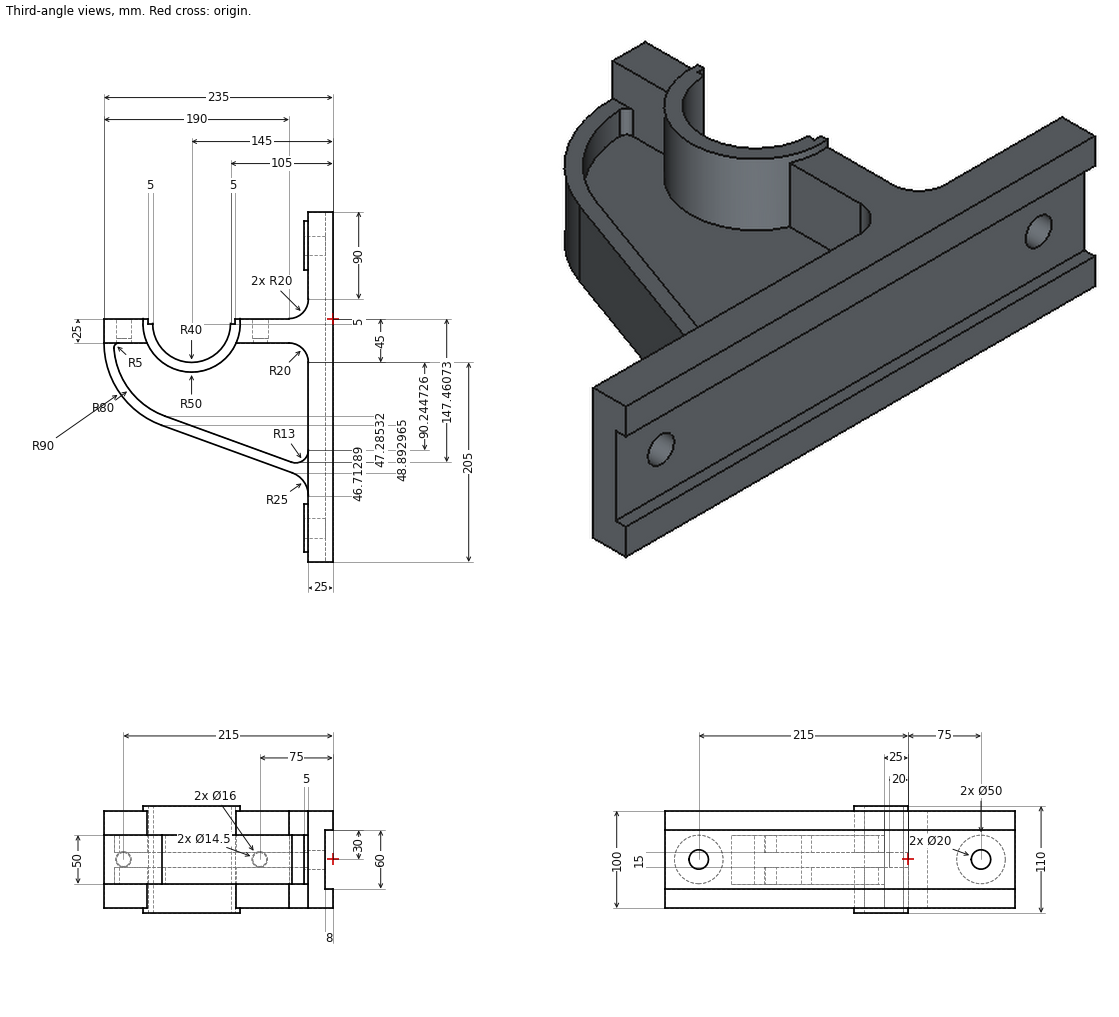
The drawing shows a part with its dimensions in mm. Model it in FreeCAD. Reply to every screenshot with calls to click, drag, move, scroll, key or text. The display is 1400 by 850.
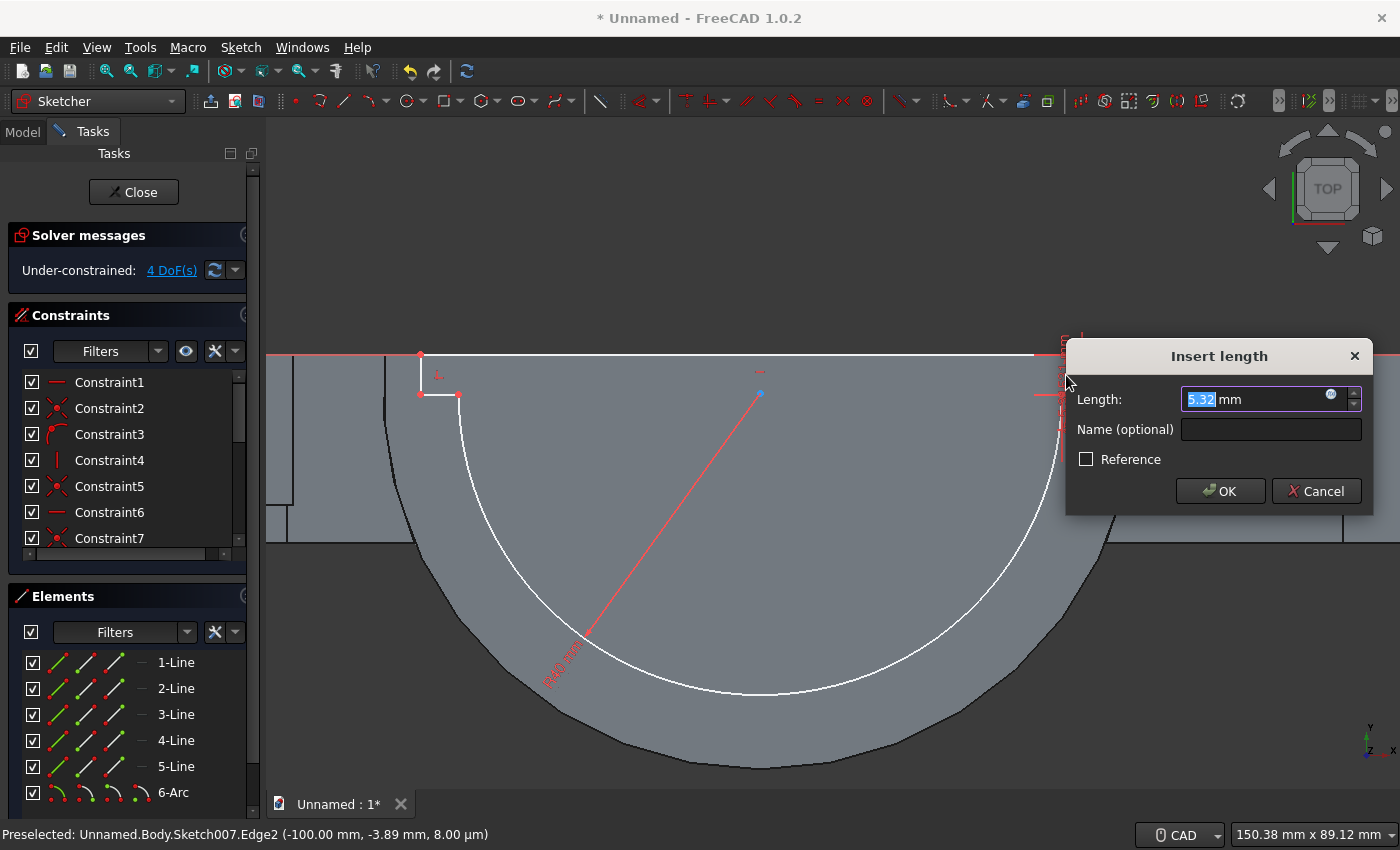
text(5)
key(Return)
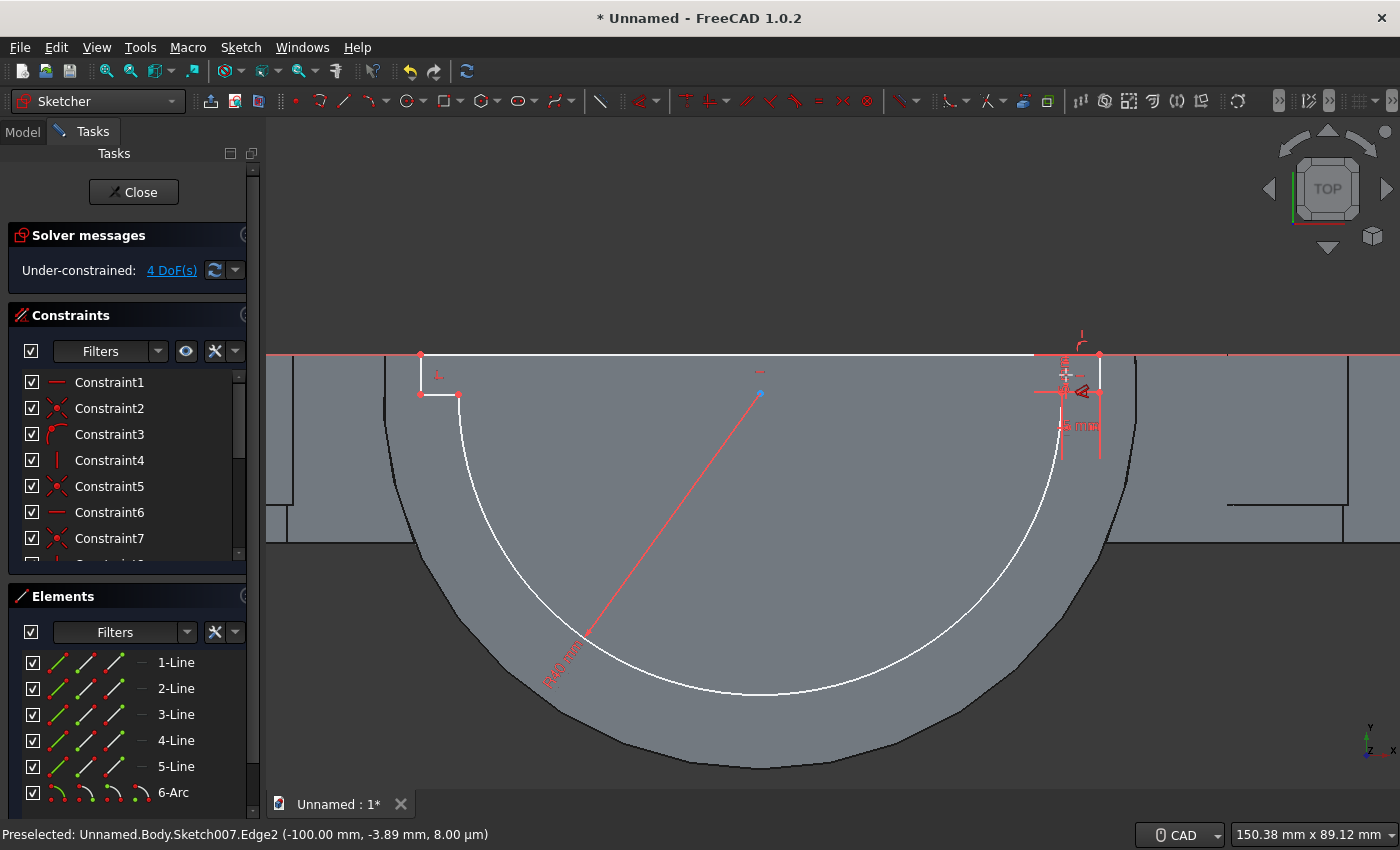
click(421, 367)
click(387, 375)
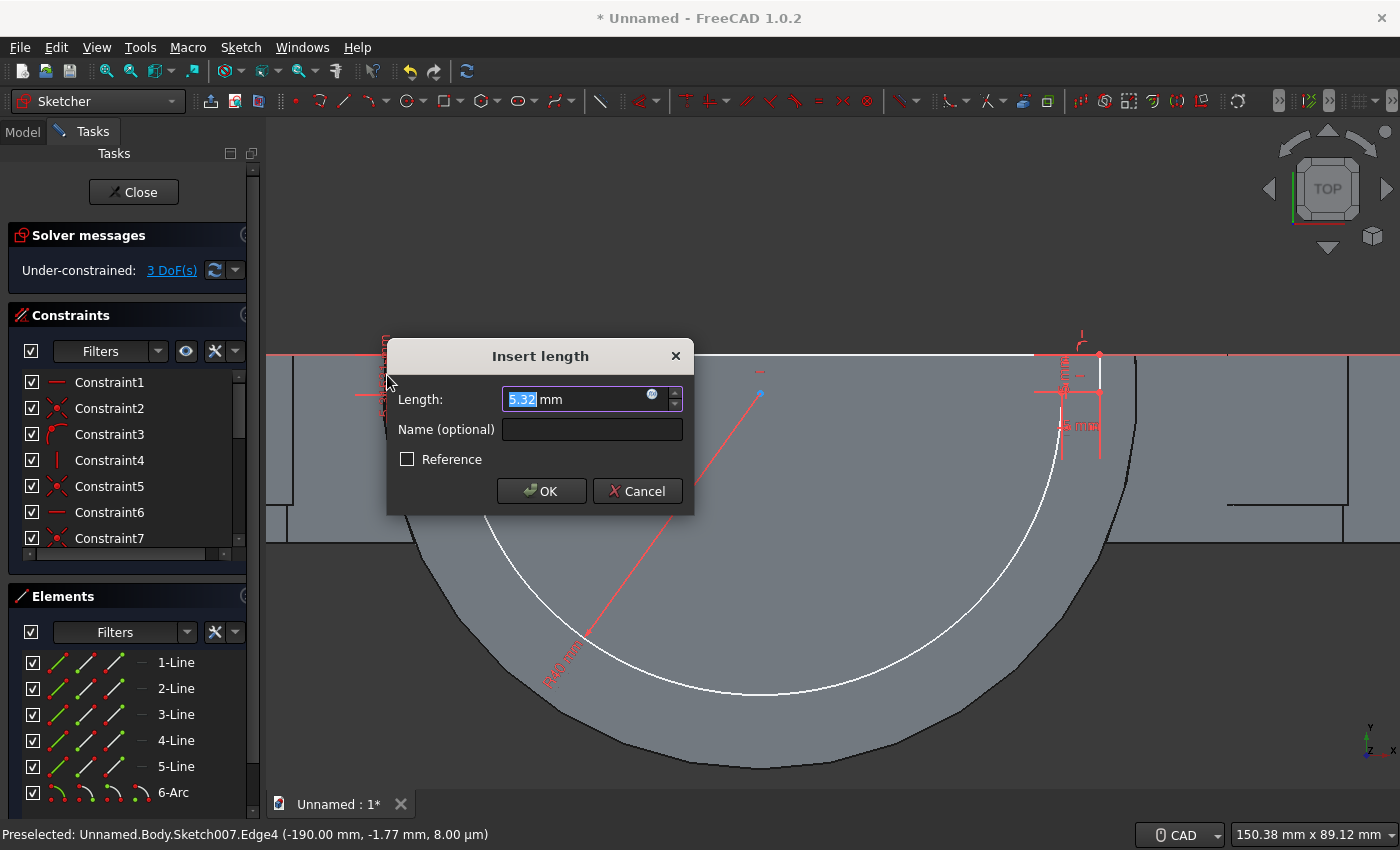
text(5)
key(Return)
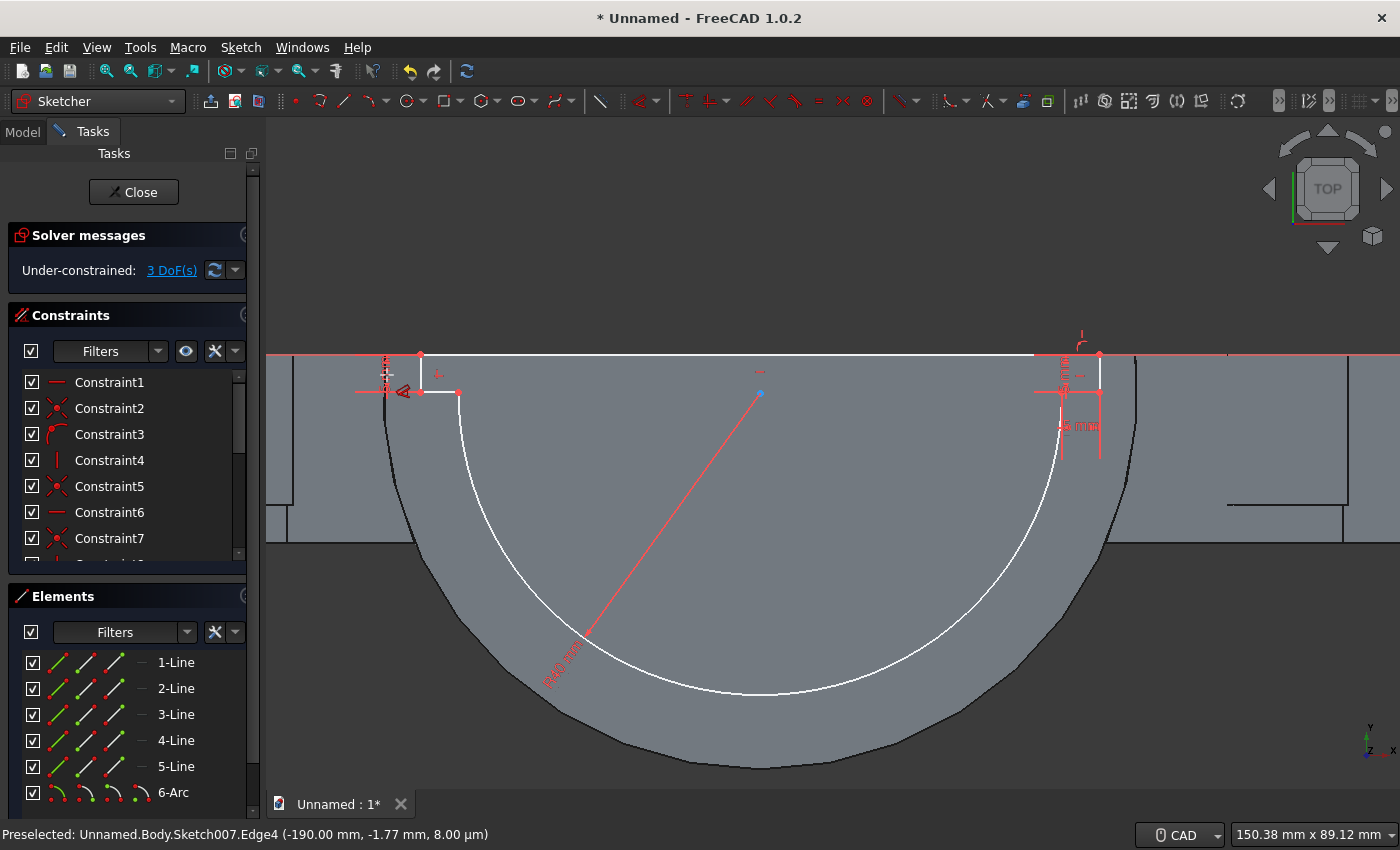
click(432, 392)
click(440, 426)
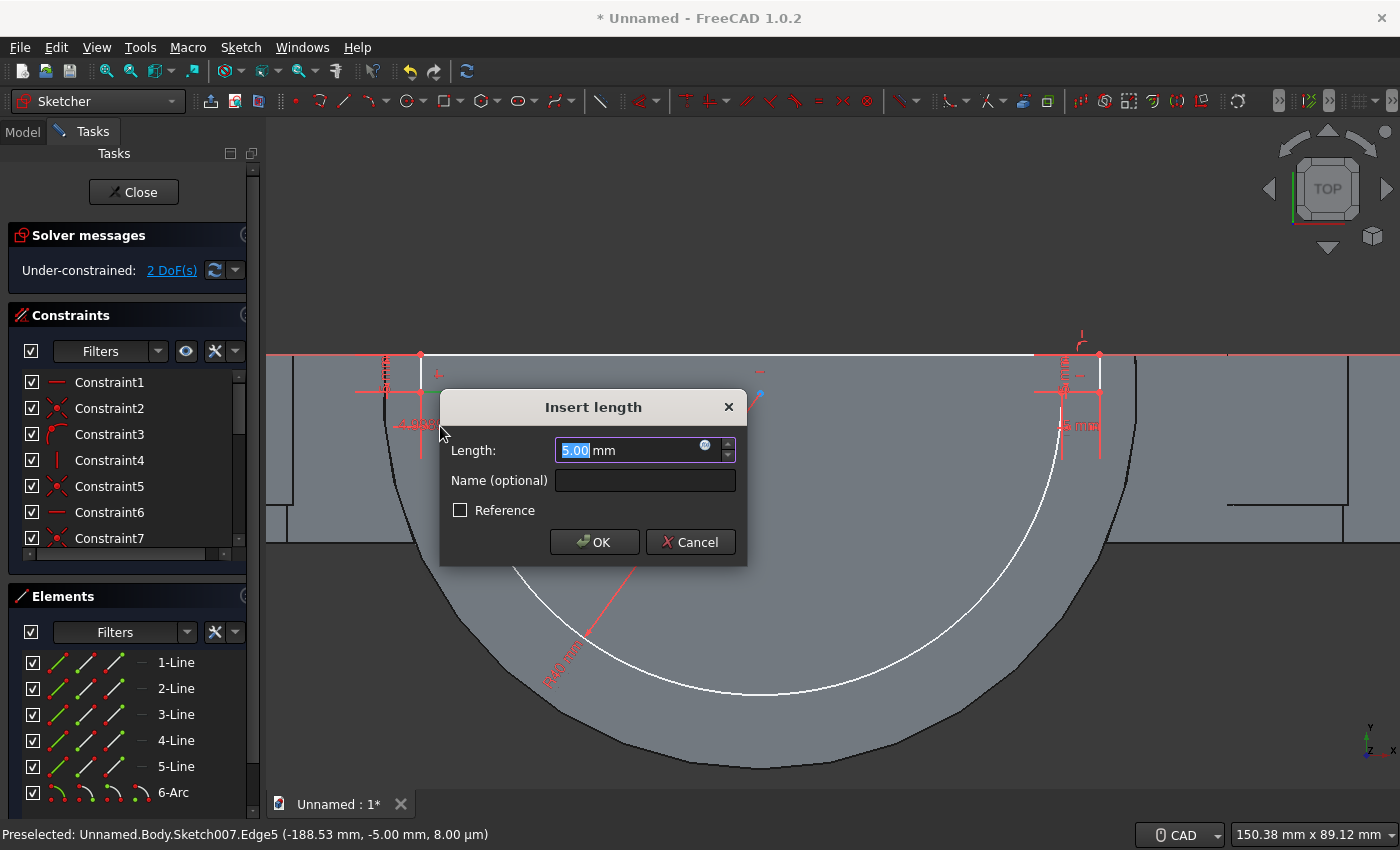
text(5)
key(Return)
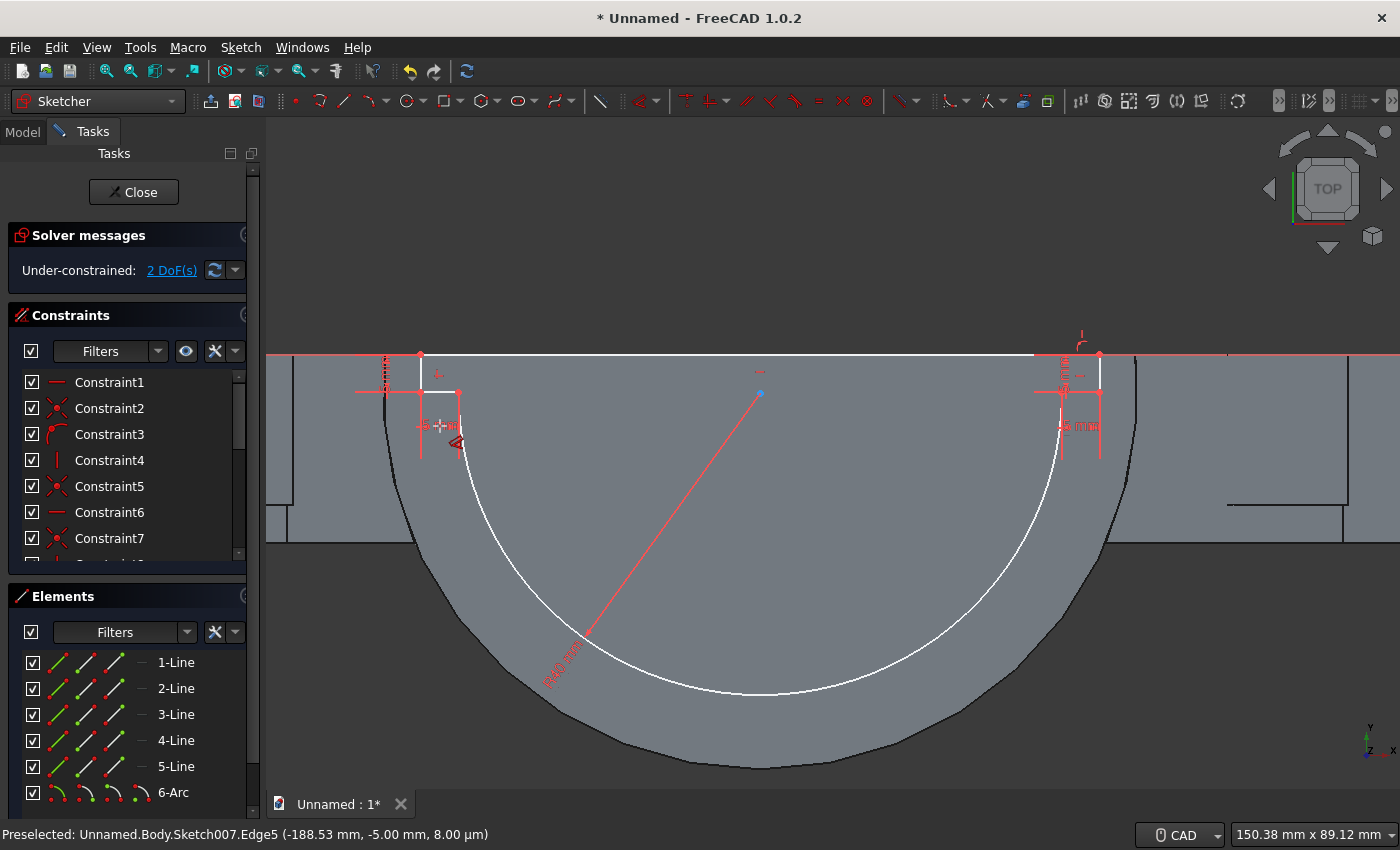
click(760, 393)
click(726, 374)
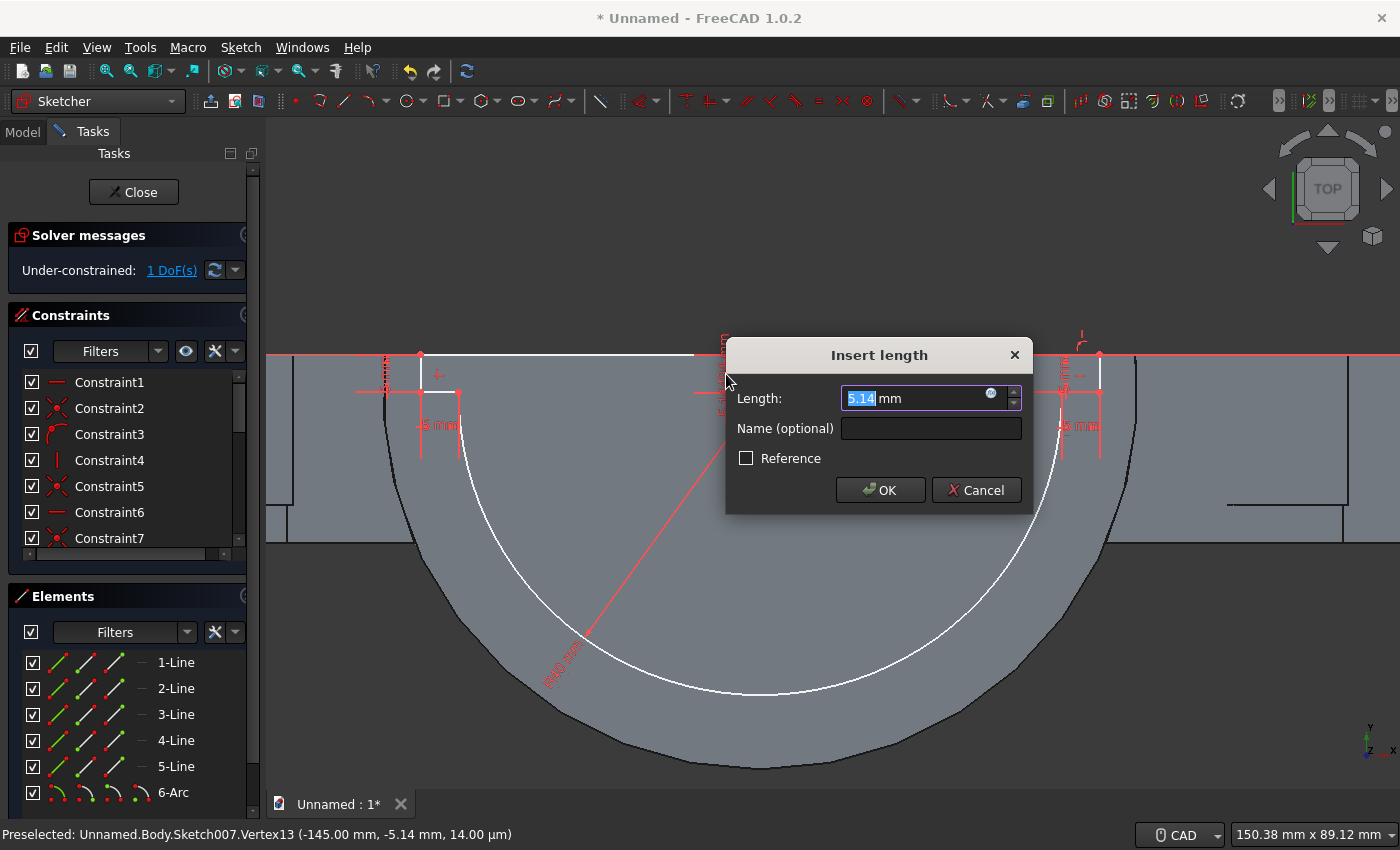
text(5)
key(Return)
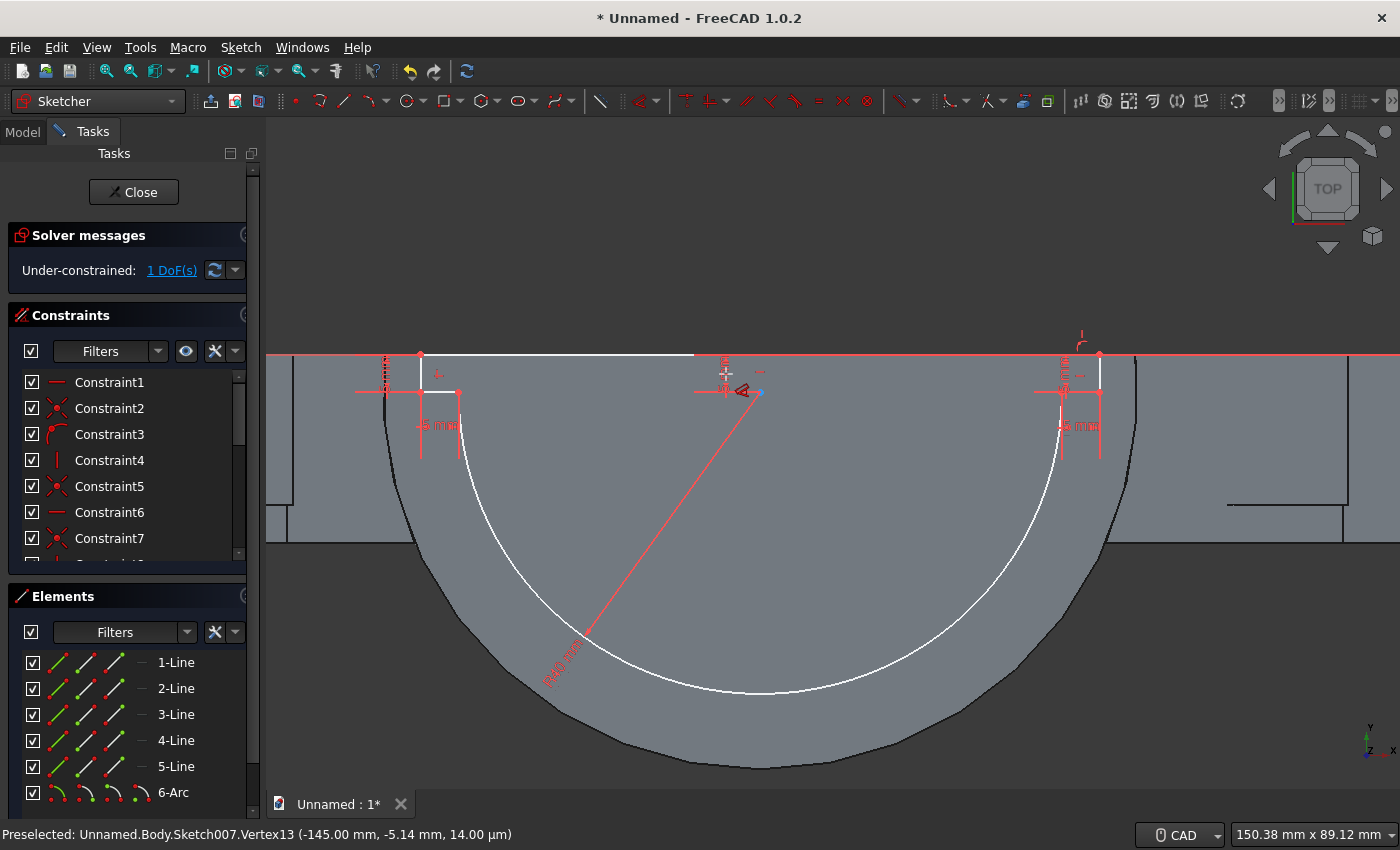
click(1062, 392)
click(1148, 321)